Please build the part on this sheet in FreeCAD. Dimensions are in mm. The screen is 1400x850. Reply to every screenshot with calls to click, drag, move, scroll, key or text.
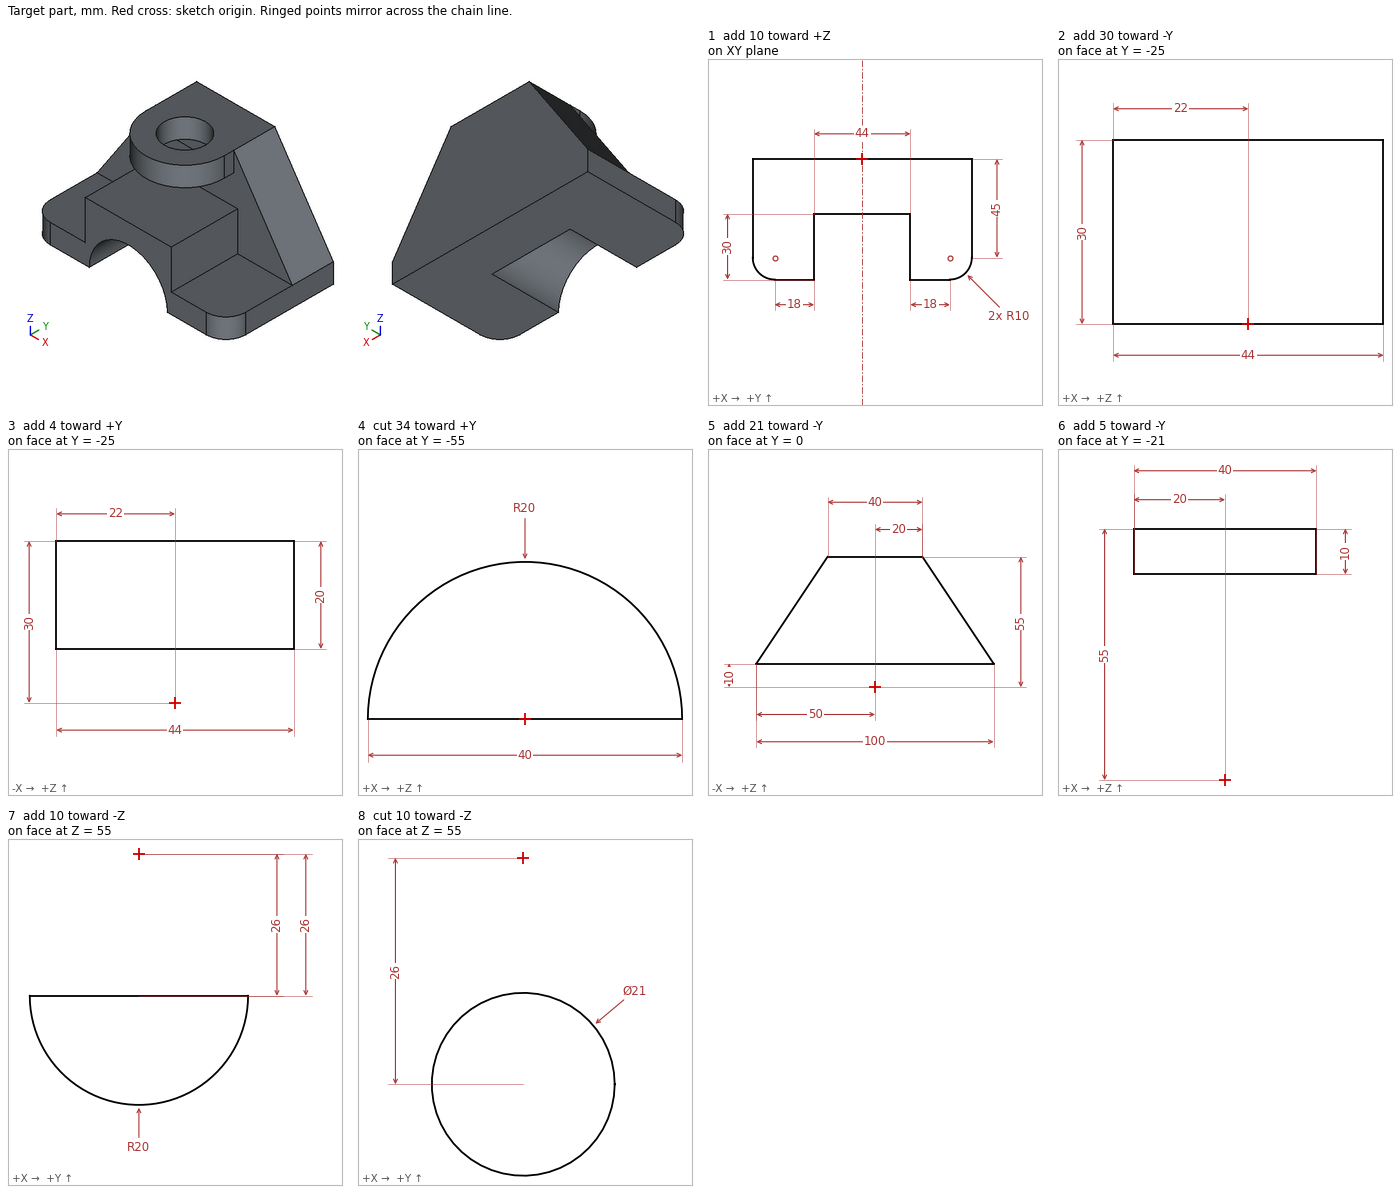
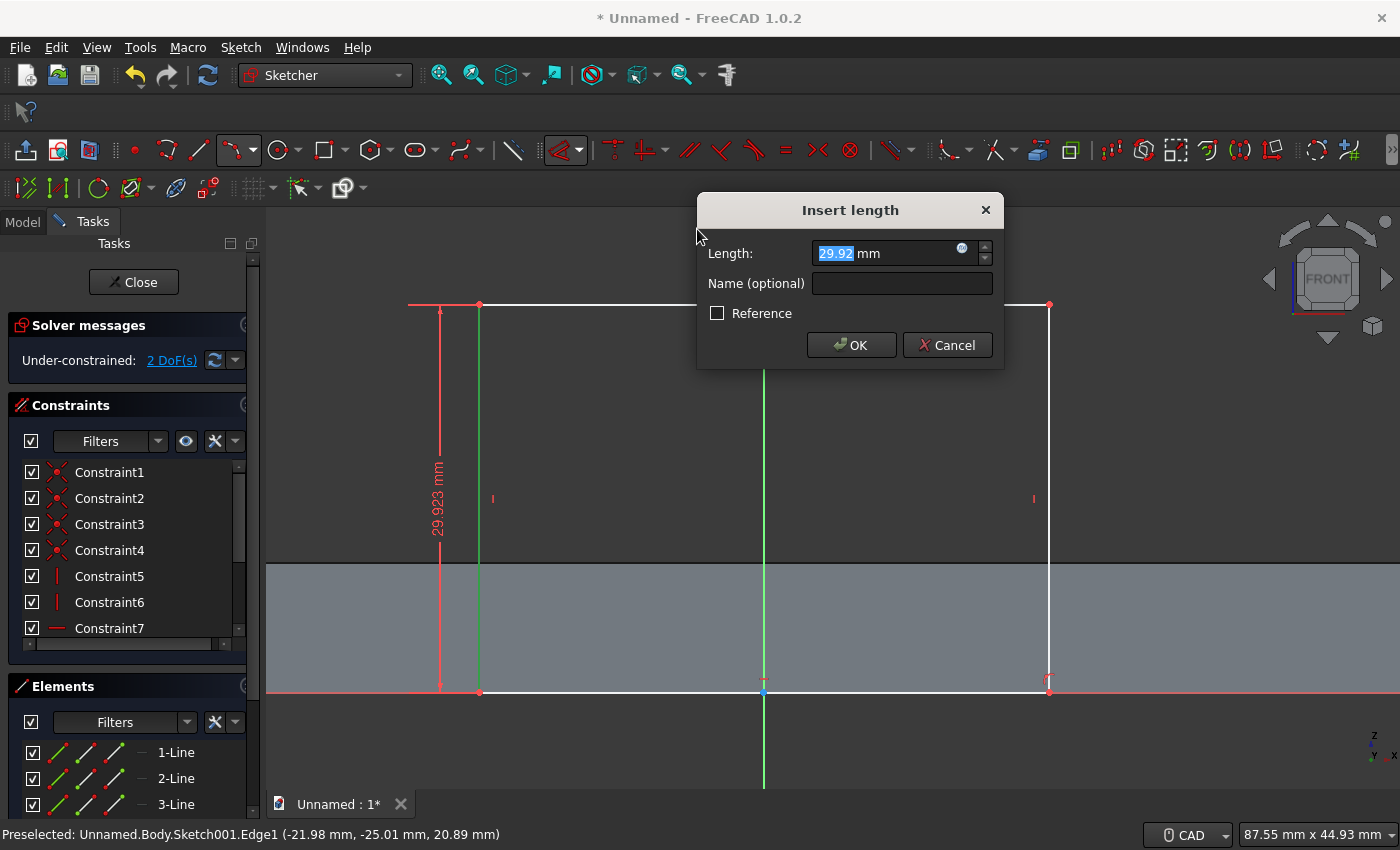
text(30)
key(Return)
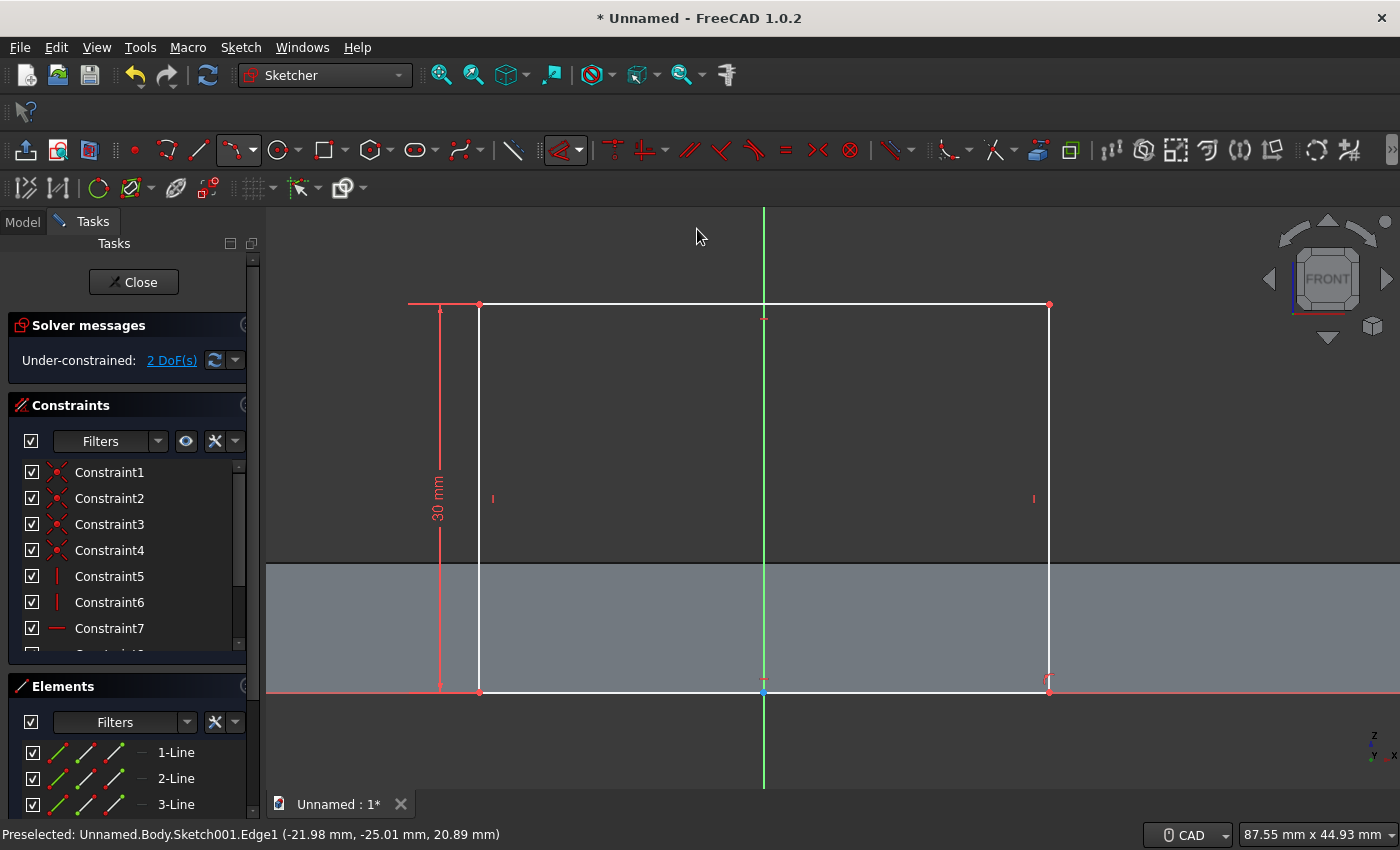
click(650, 693)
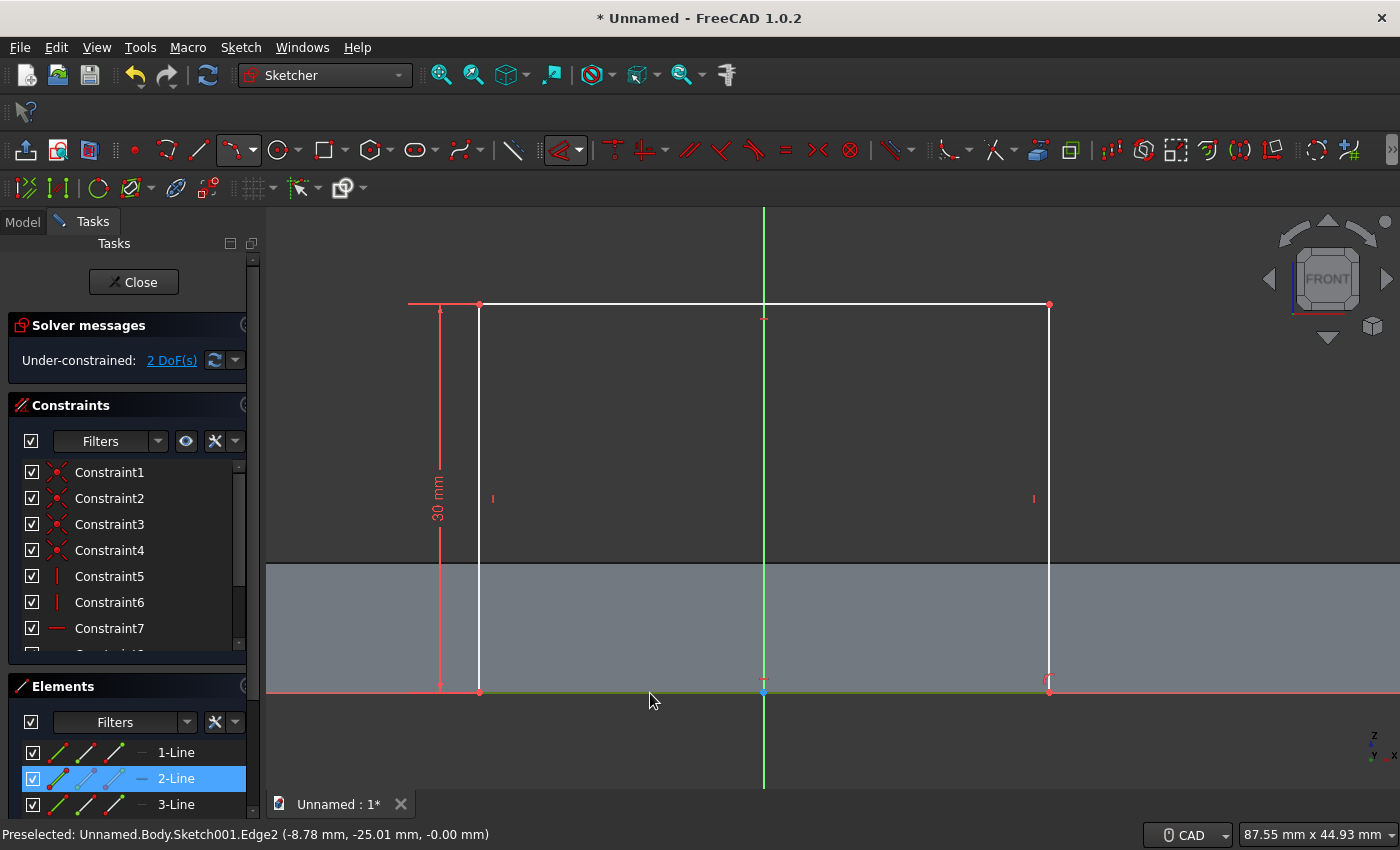
key(l)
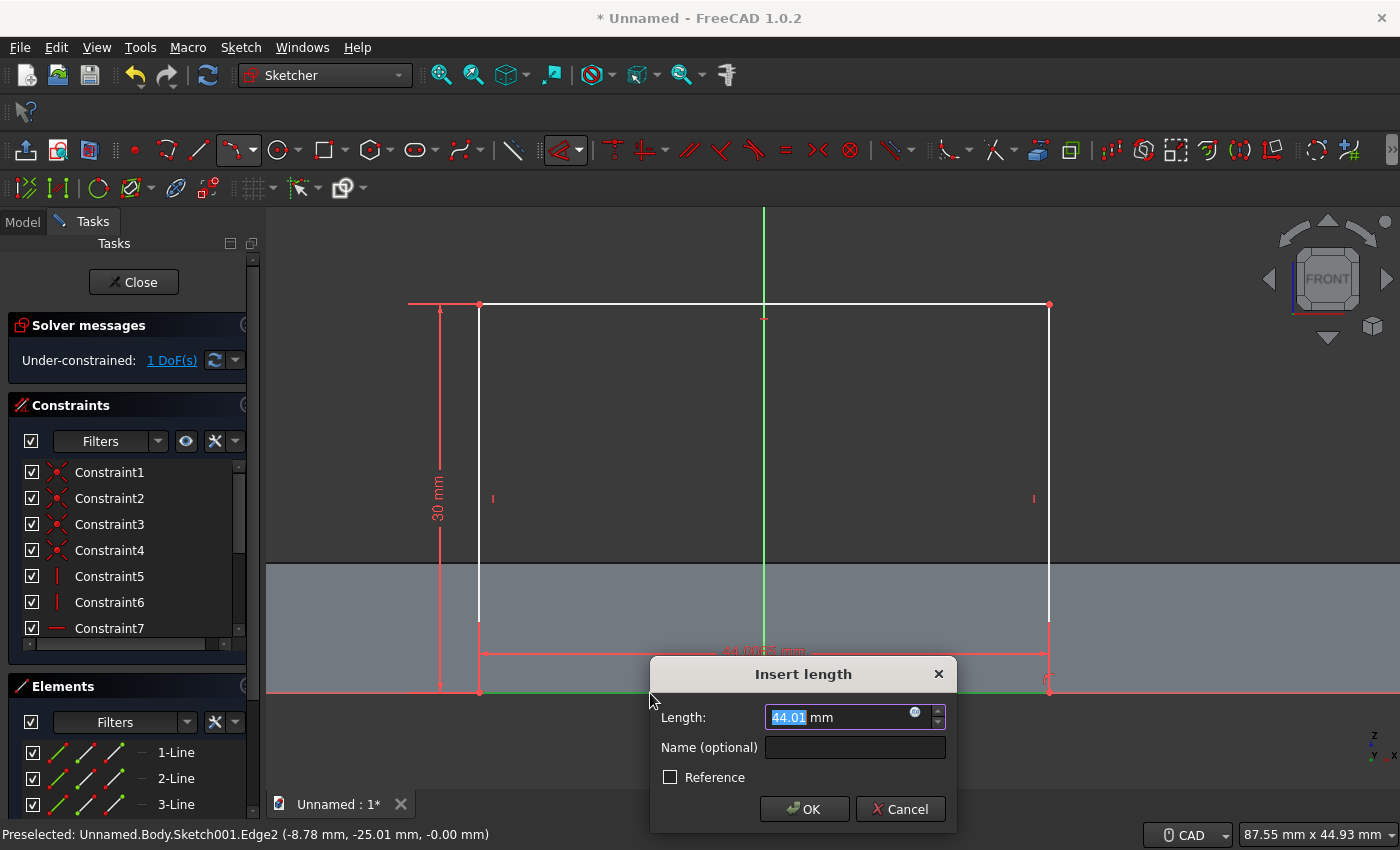
text(44)
key(Return)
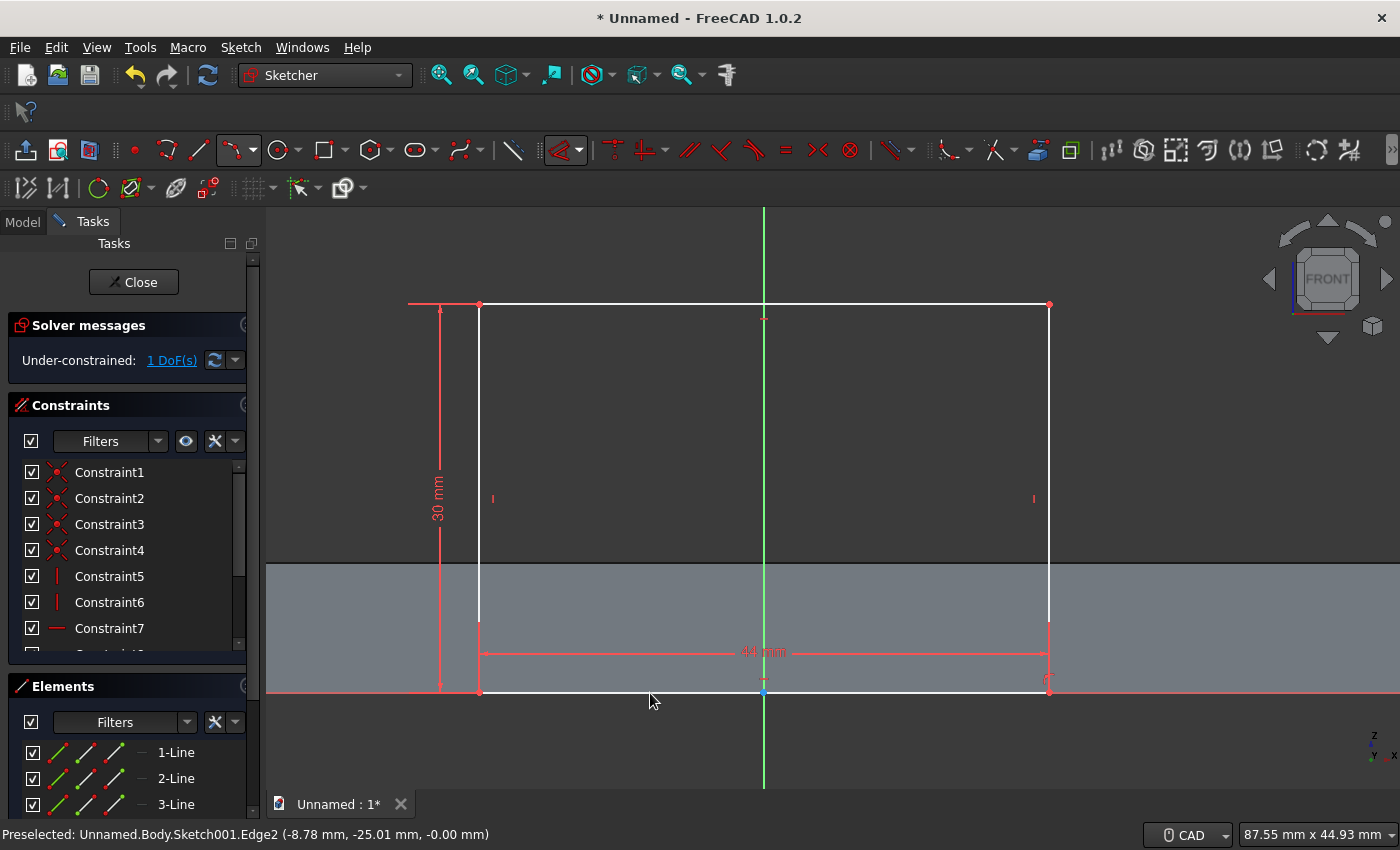
click(479, 304)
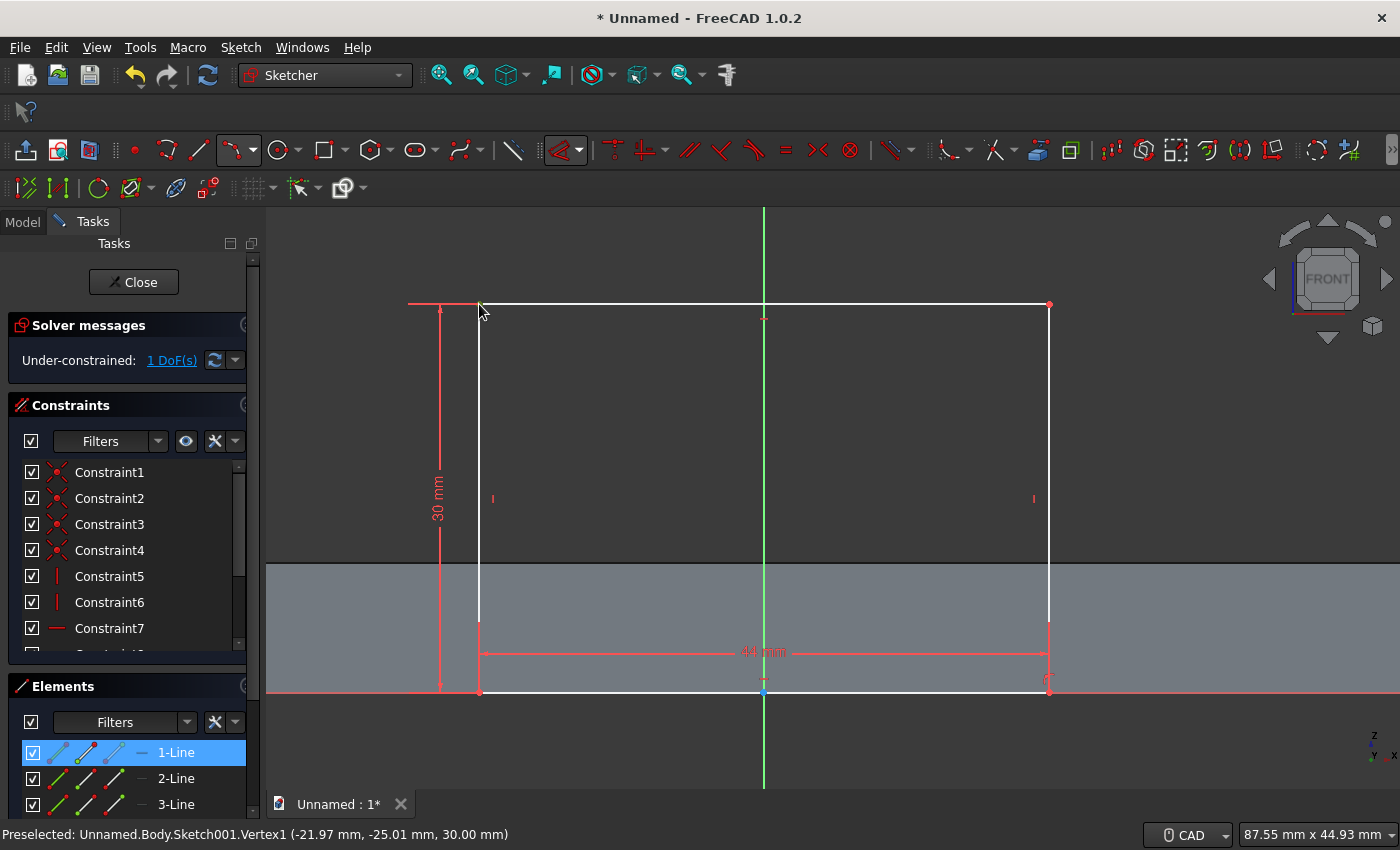
click(582, 150)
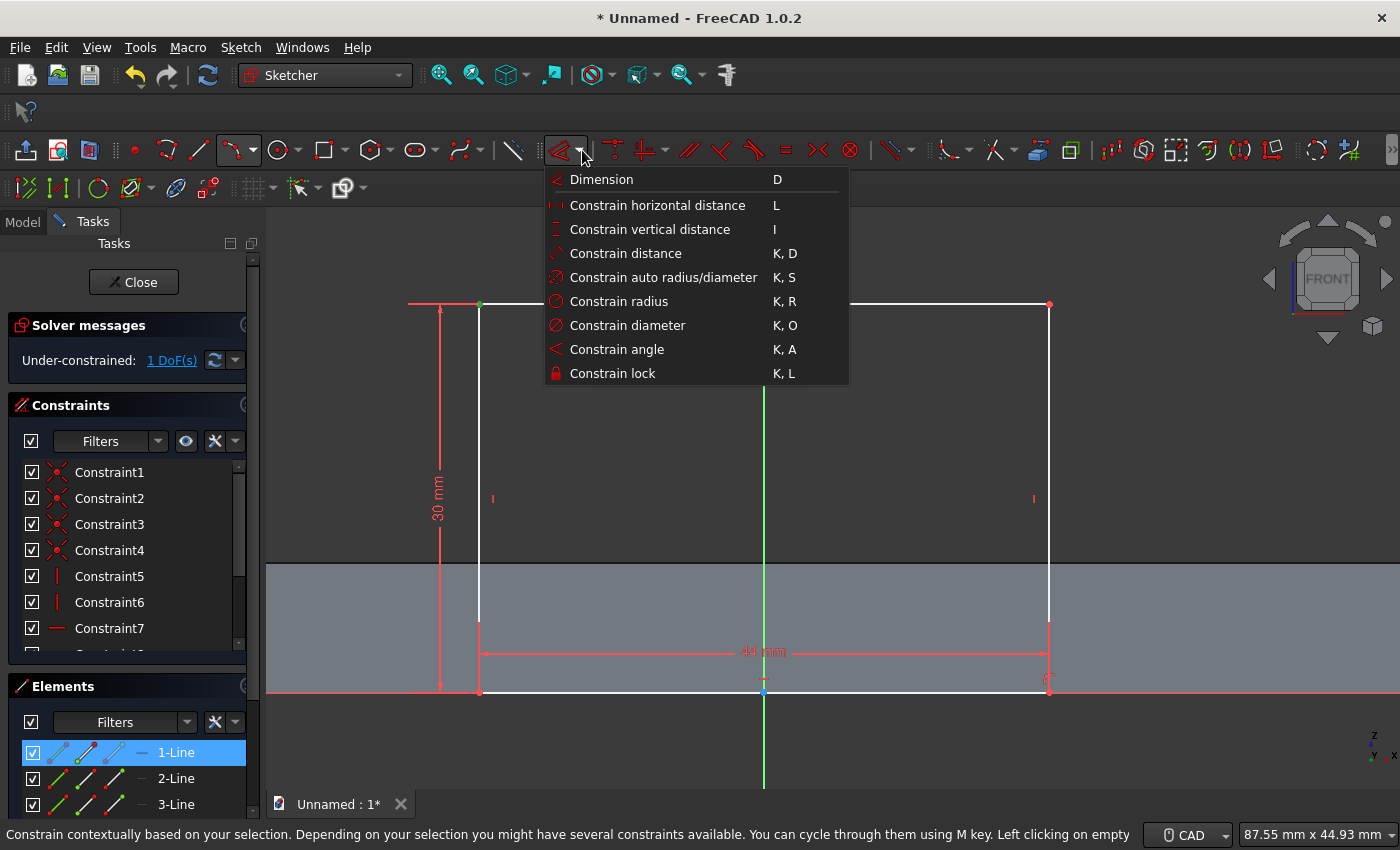
click(697, 205)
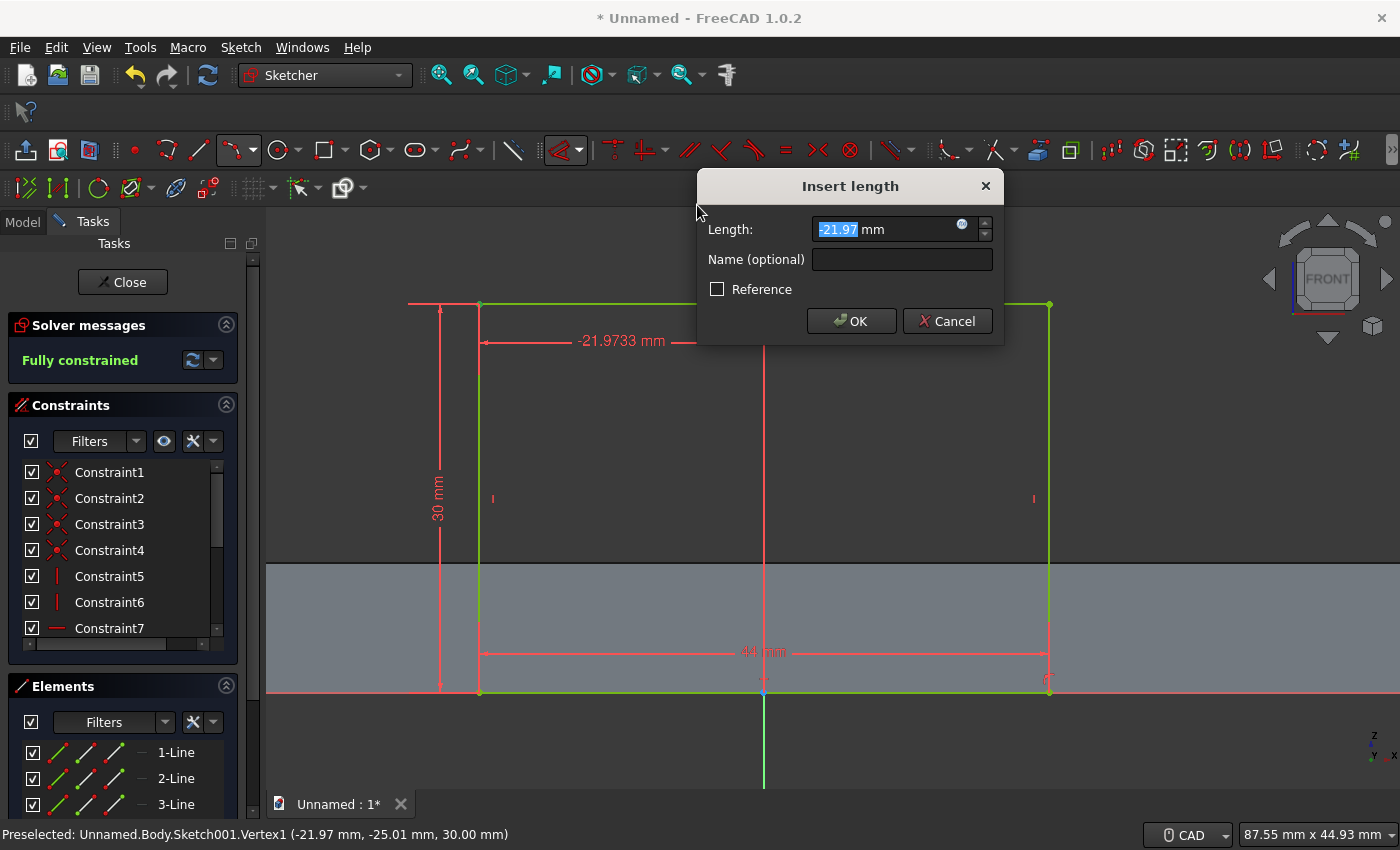
text(-22)
key(Return)